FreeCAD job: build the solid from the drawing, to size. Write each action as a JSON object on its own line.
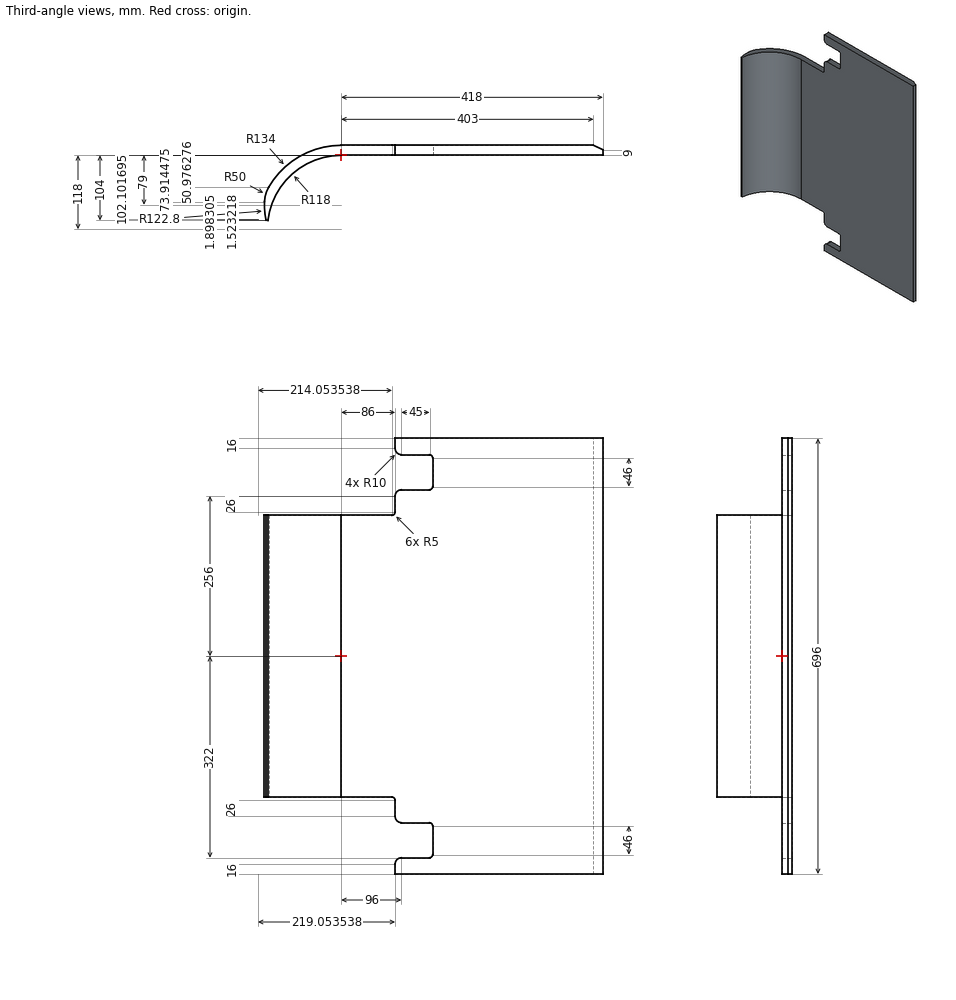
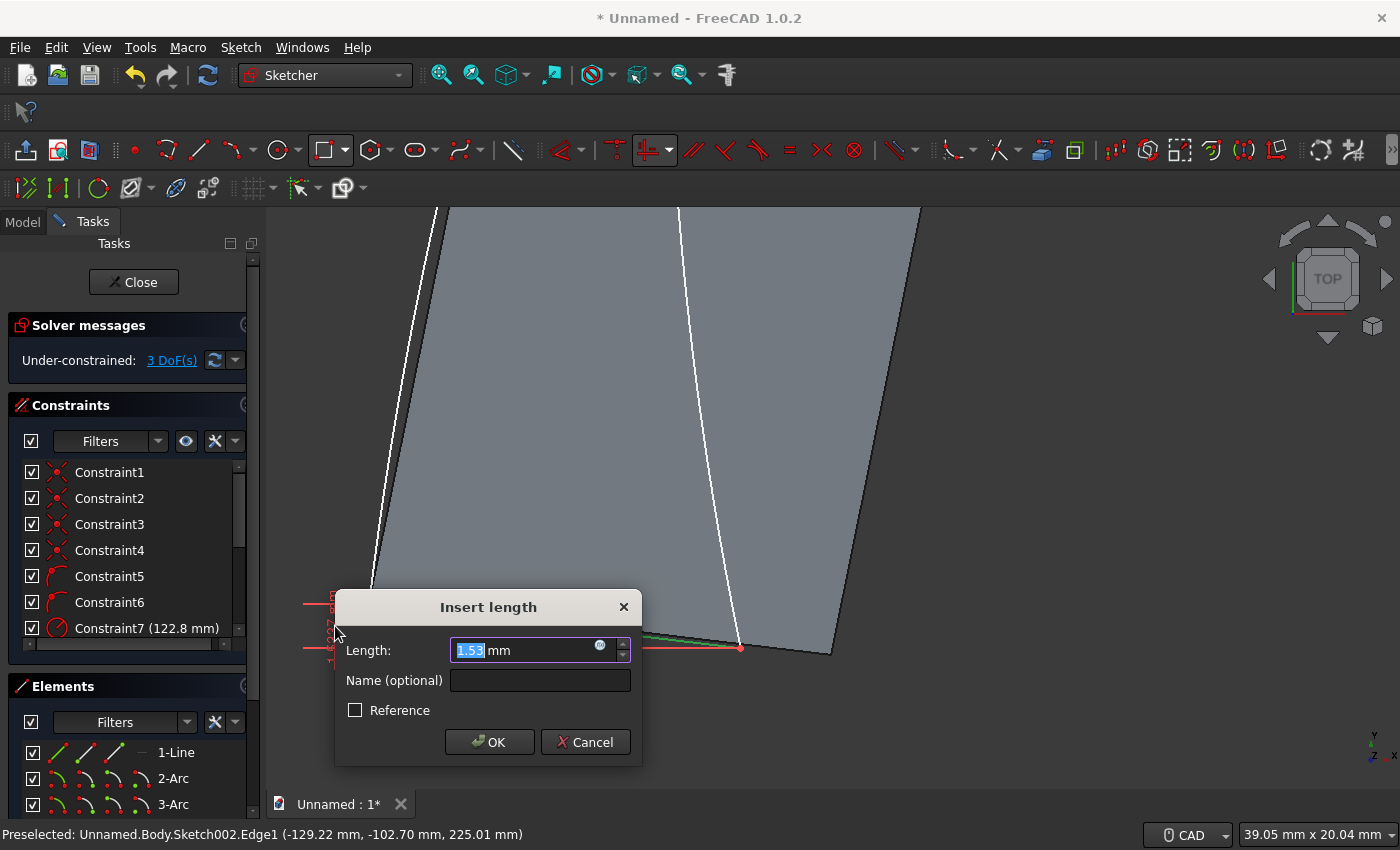
{"action": "type", "text": "1.523218"}
{"action": "key", "text": "Return"}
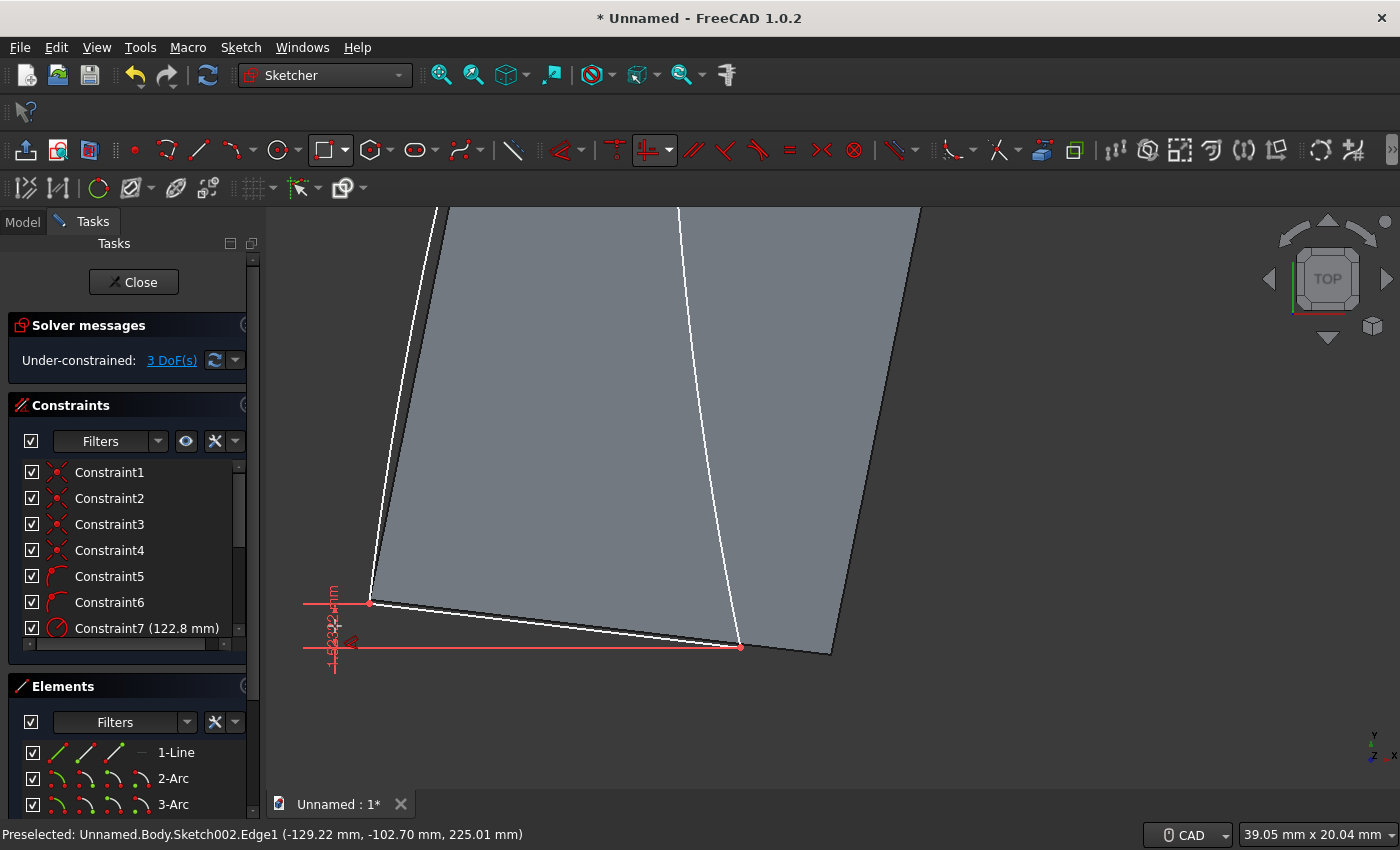
{"action": "scroll", "coordinate": [813, 700], "scroll_direction": "down", "scroll_amount": 7}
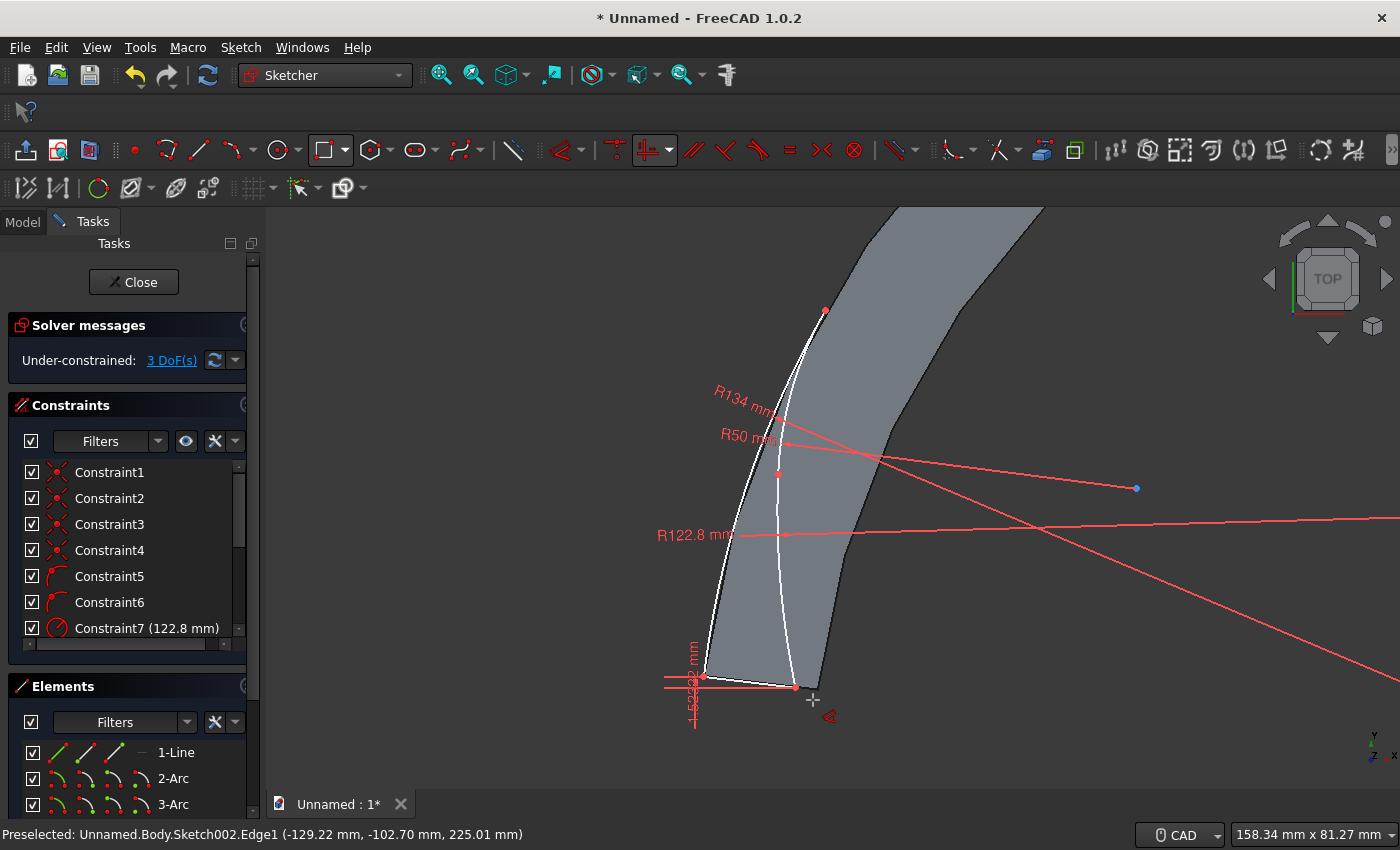
{"action": "left_click", "coordinate": [778, 475]}
{"action": "left_click", "coordinate": [744, 355]}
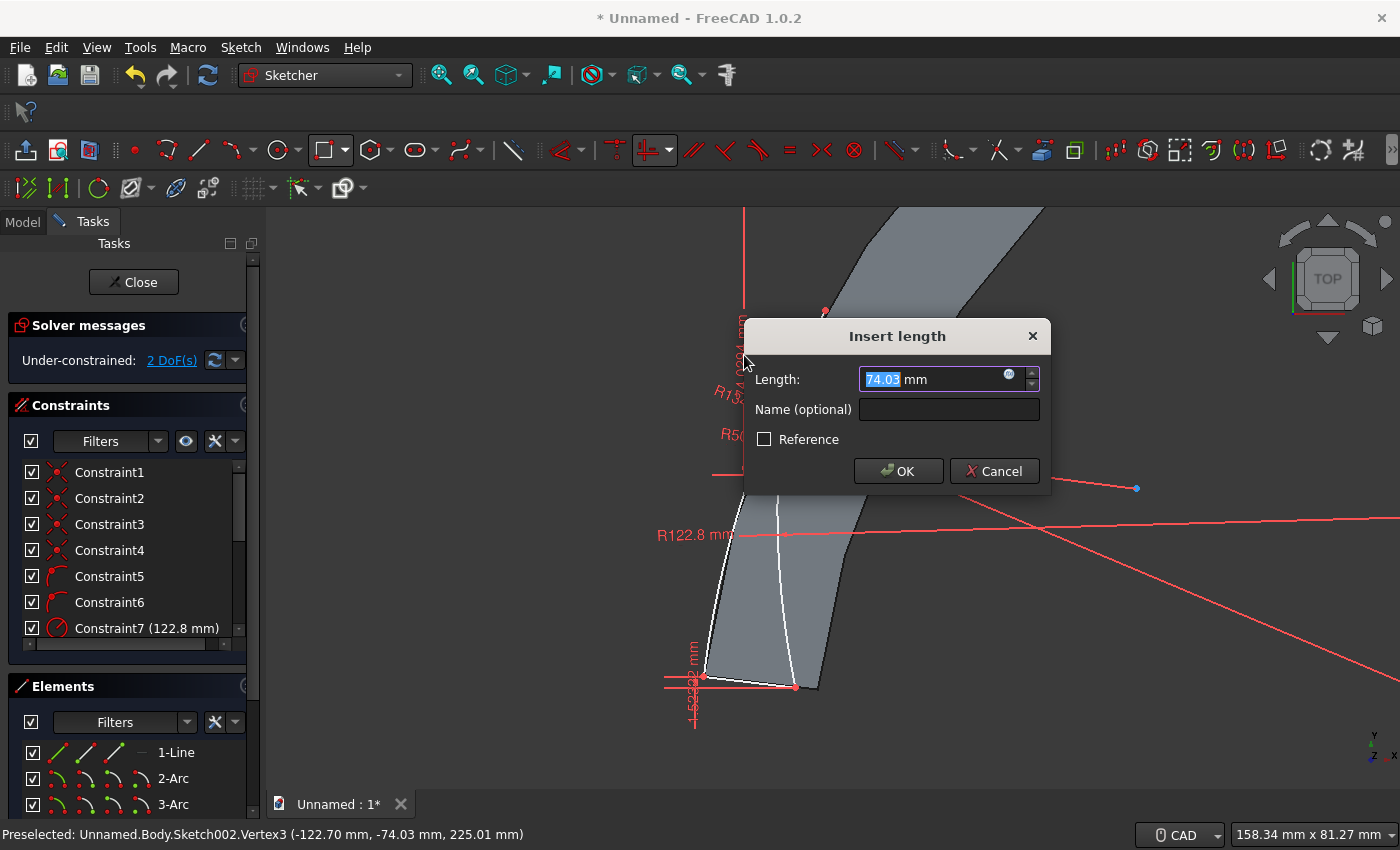
{"action": "type", "text": "73.914475"}
{"action": "key", "text": "Return"}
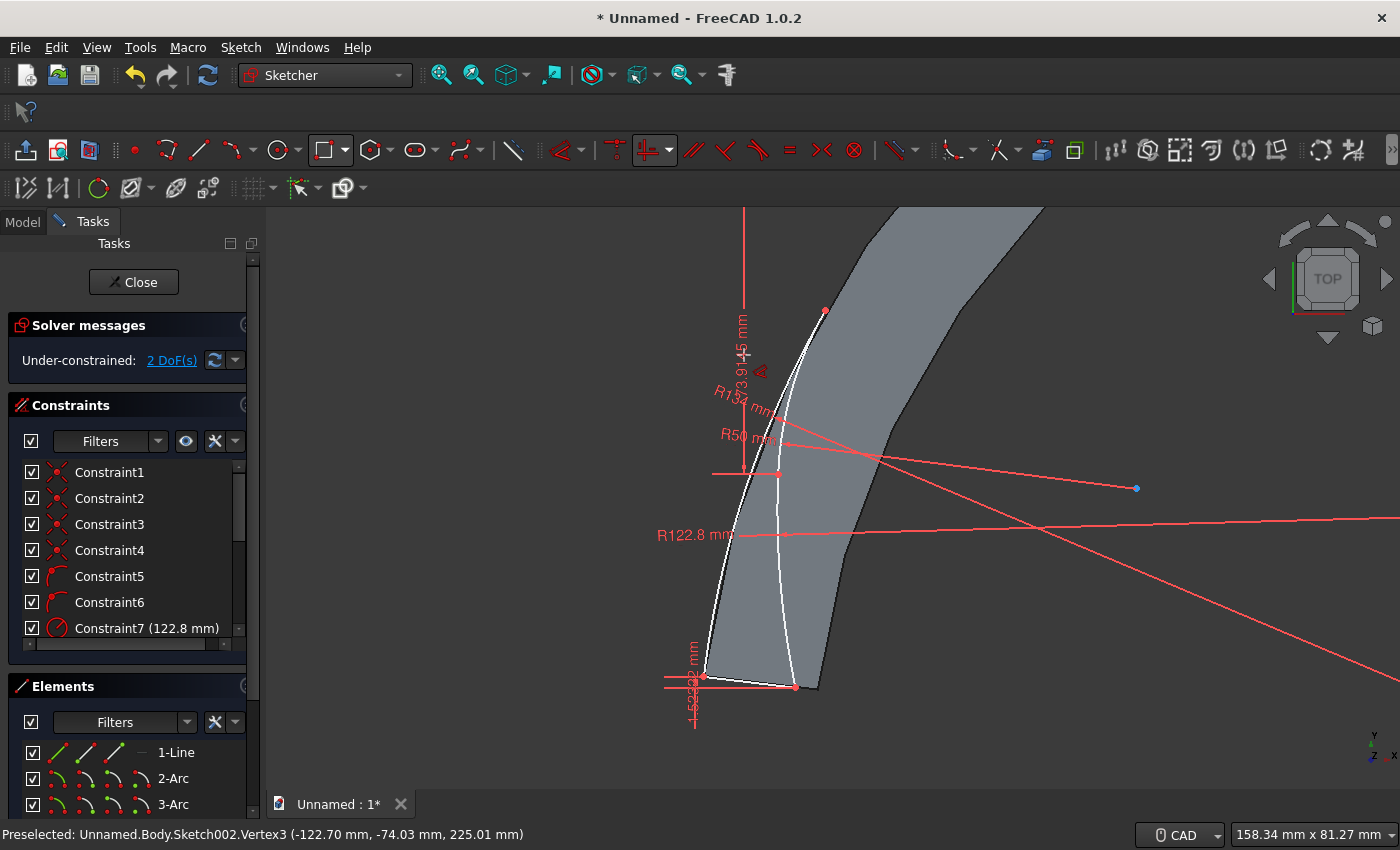
{"action": "left_click", "coordinate": [825, 311]}
{"action": "left_click", "coordinate": [791, 273]}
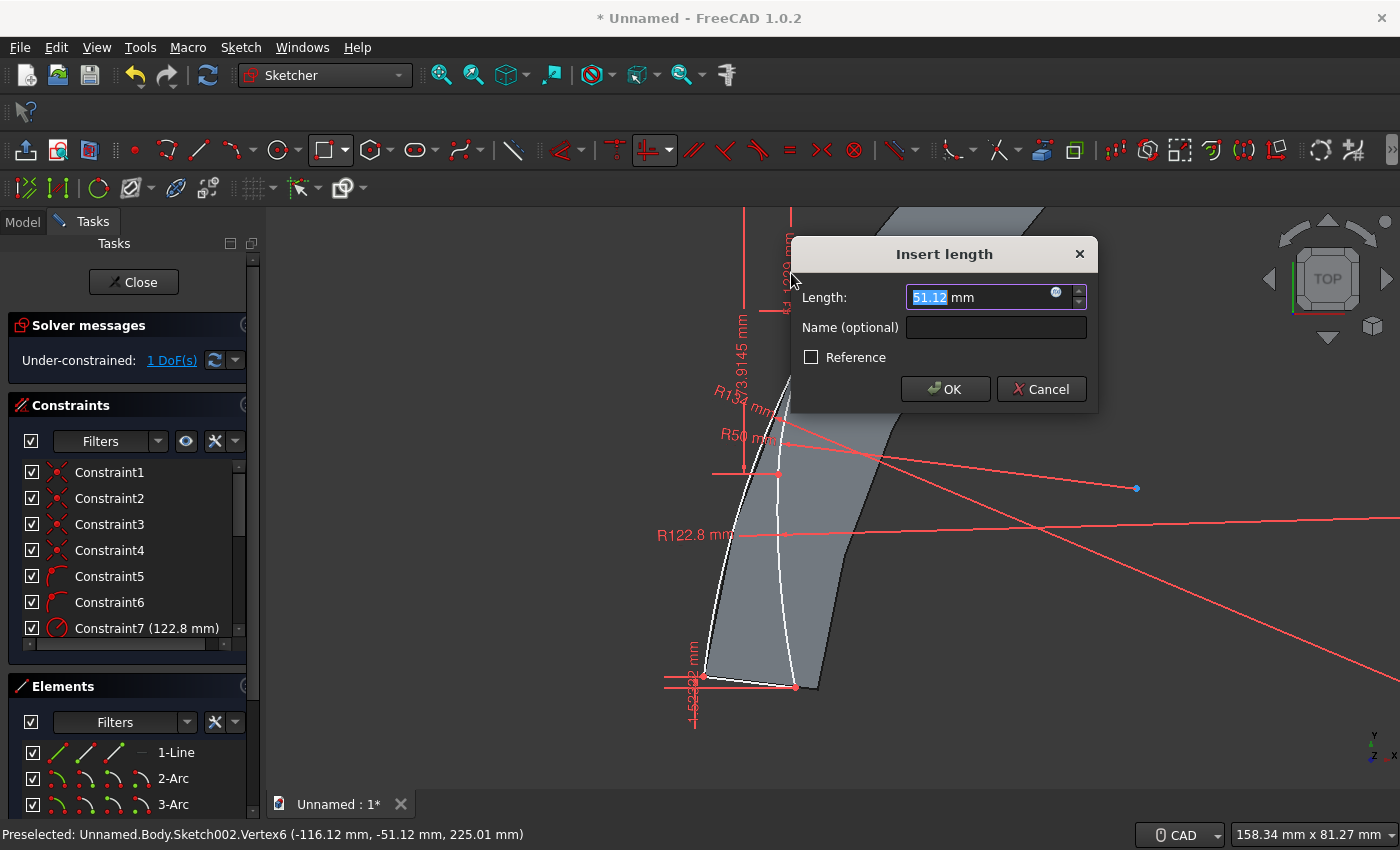
{"action": "type", "text": "50.976276"}
{"action": "key", "text": "Return"}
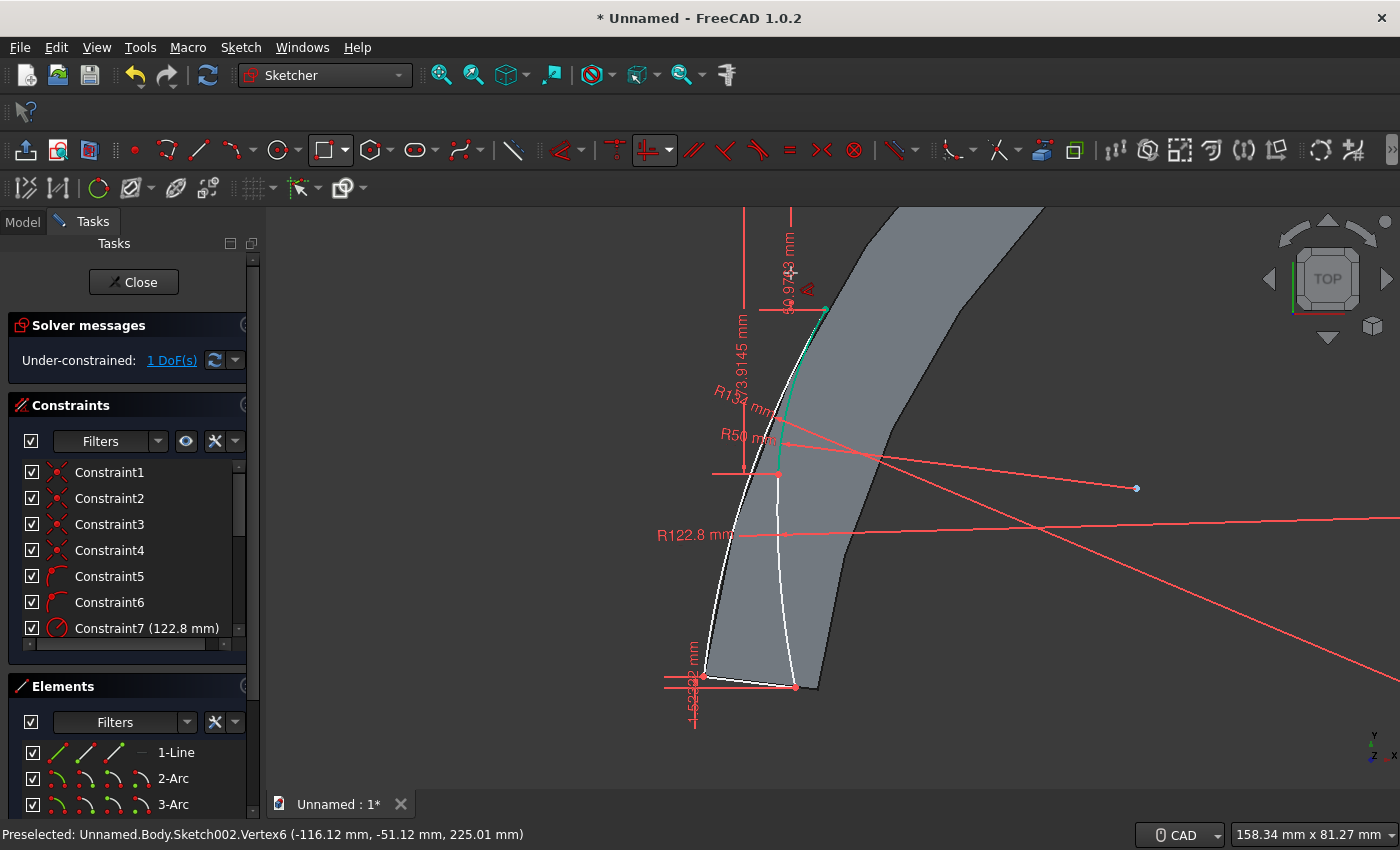
{"action": "left_click", "coordinate": [704, 677]}
{"action": "left_click", "coordinate": [670, 456]}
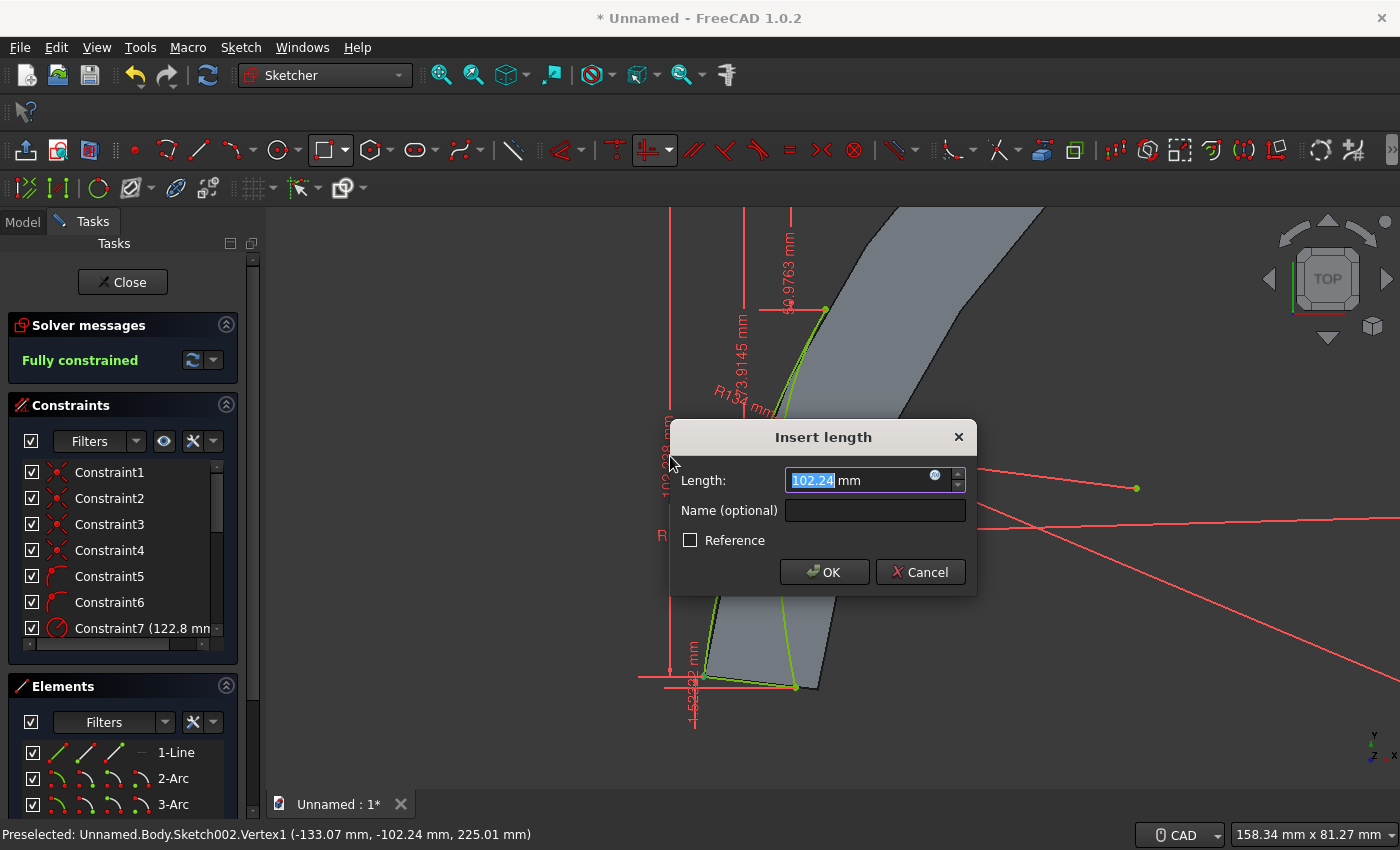
{"action": "type", "text": "102.101695"}
{"action": "key", "text": "Return"}
{"action": "key", "text": "Escape"}